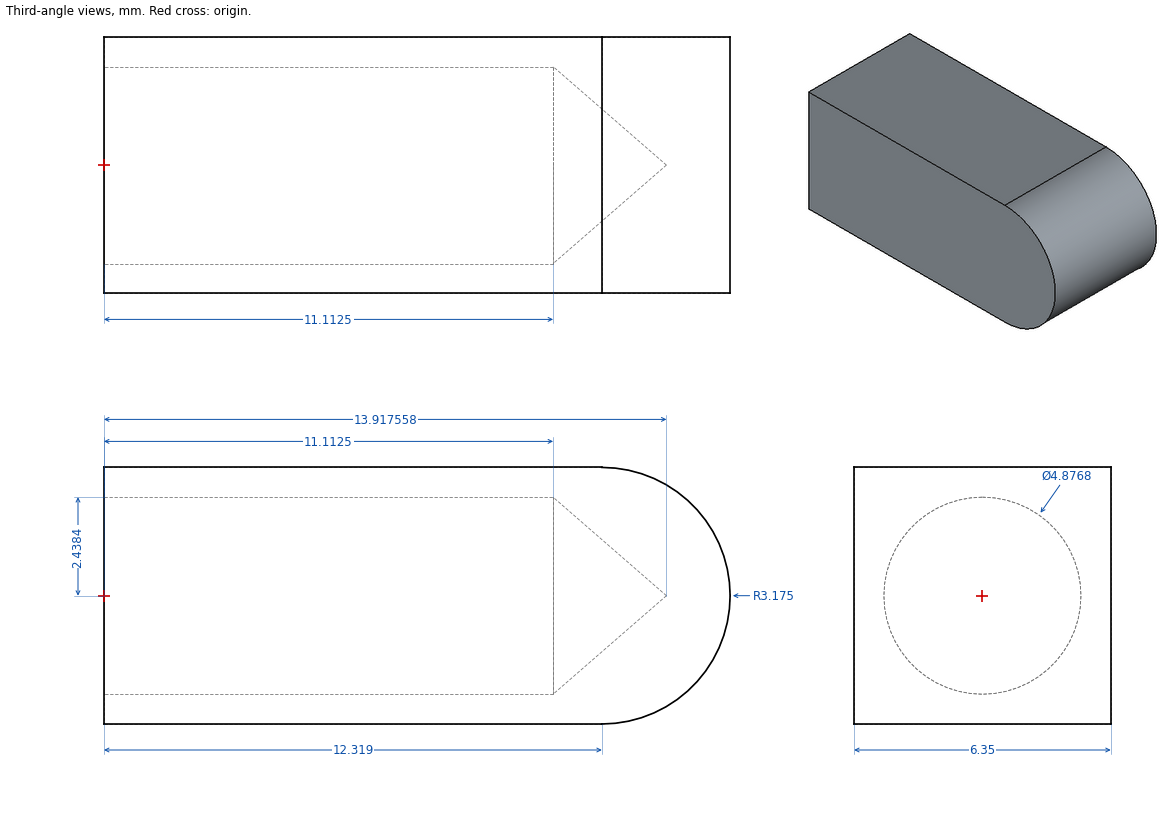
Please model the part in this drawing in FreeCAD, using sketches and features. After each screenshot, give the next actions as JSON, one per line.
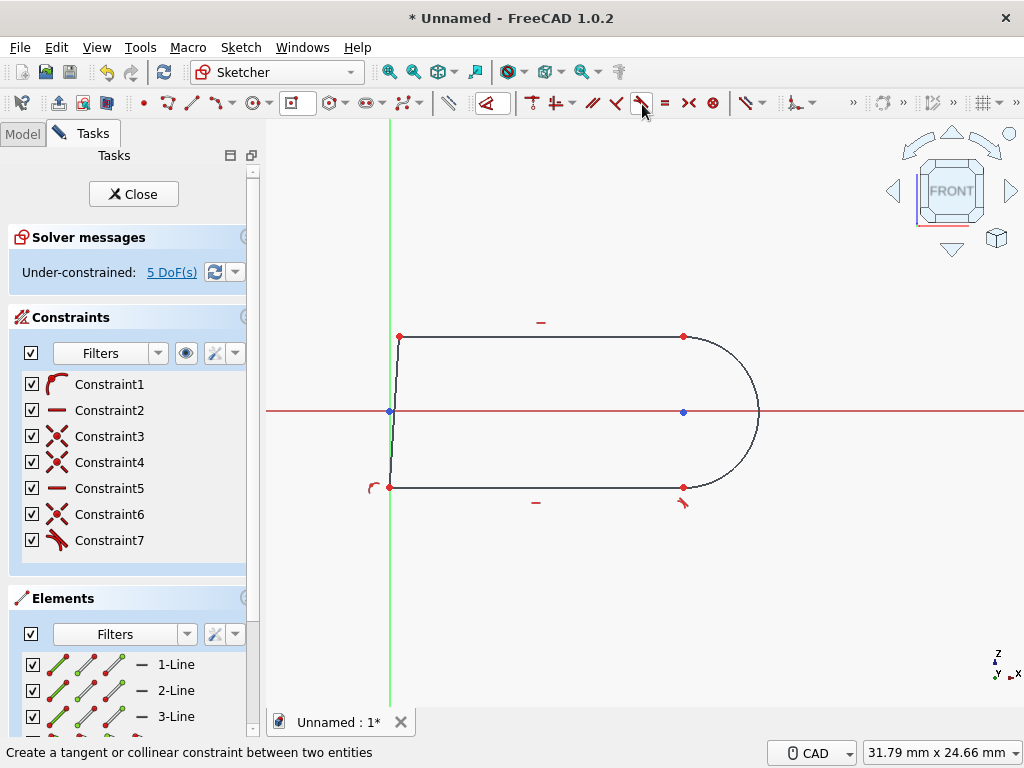
{"action": "left_click", "coordinate": [484, 337]}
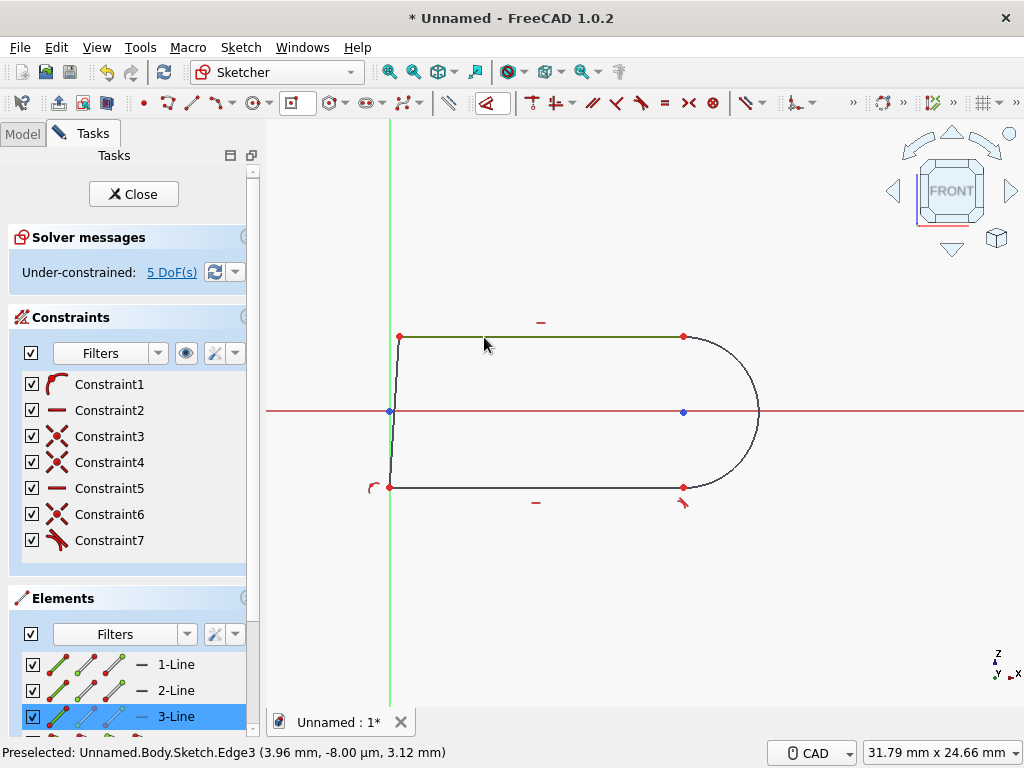
{"action": "left_click", "coordinate": [744, 457]}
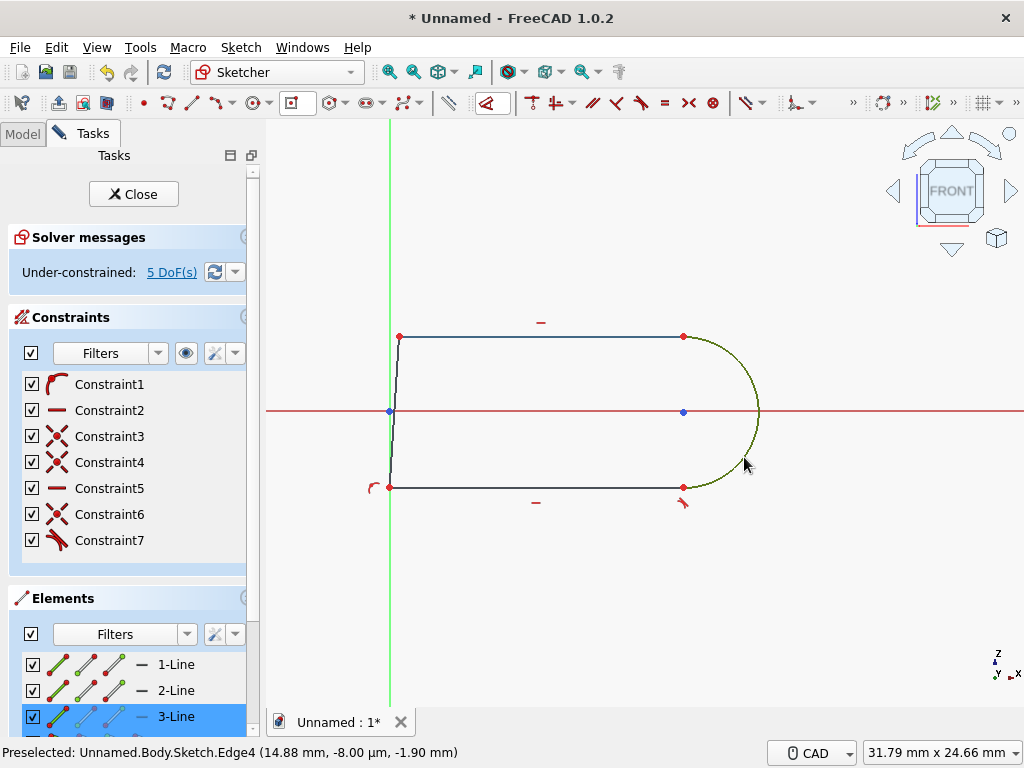
{"action": "key", "text": "t"}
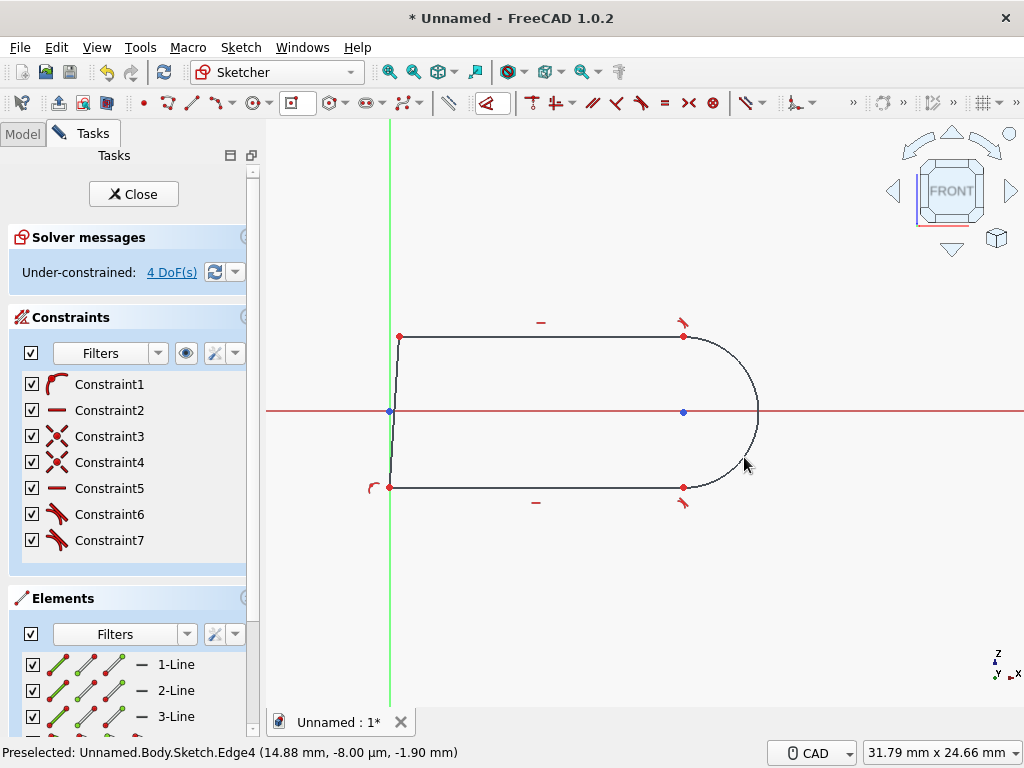
{"action": "left_click", "coordinate": [392, 443]}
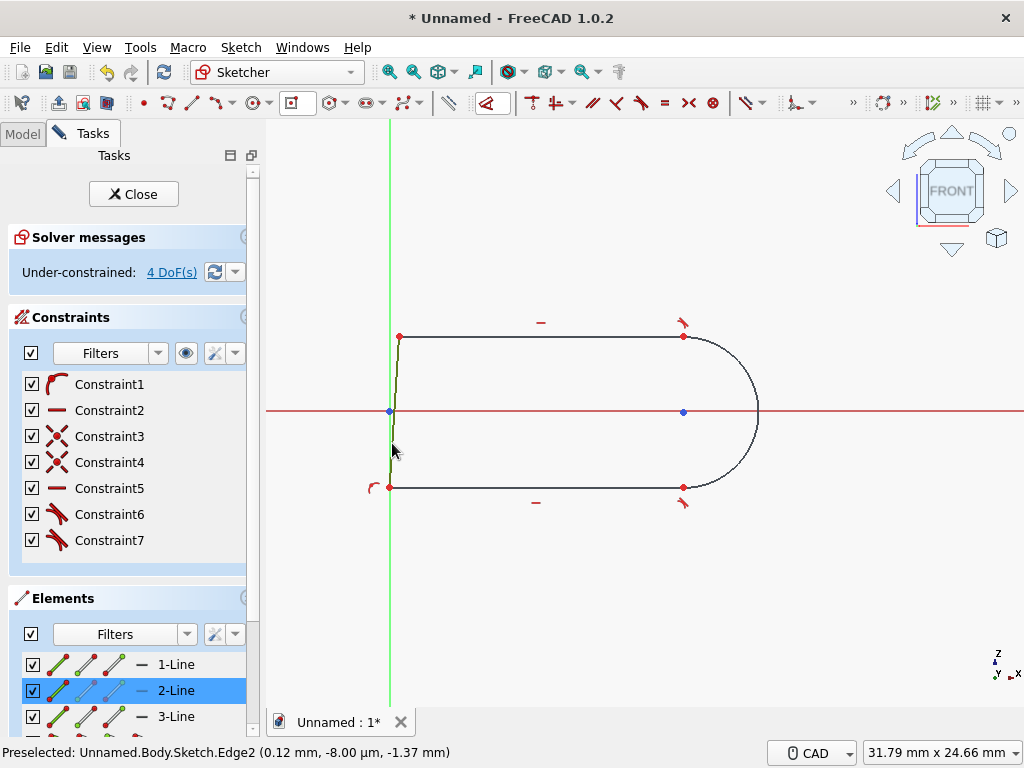
{"action": "key", "text": "v"}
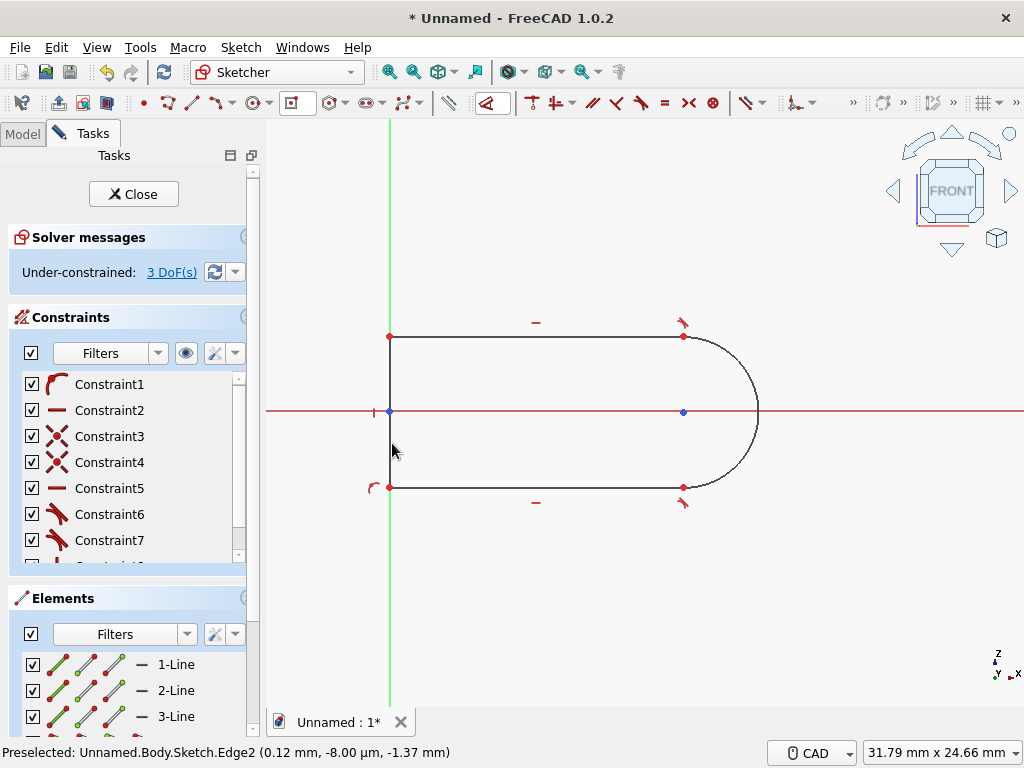
{"action": "left_click", "coordinate": [683, 412]}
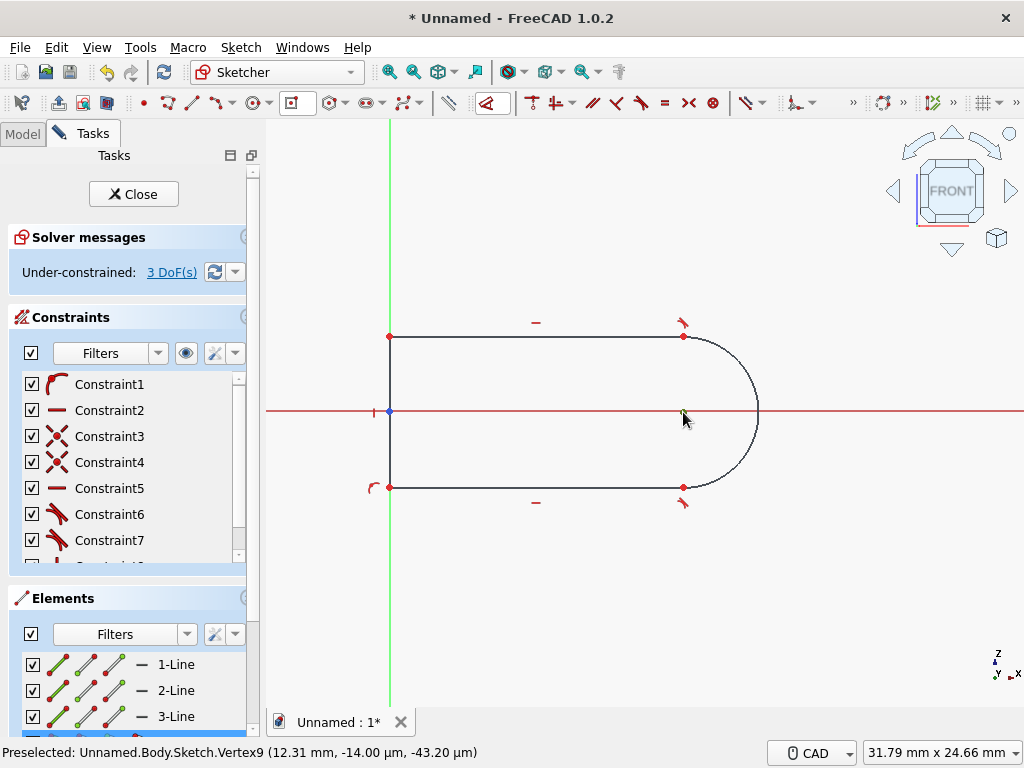
{"action": "left_click", "coordinate": [334, 411]}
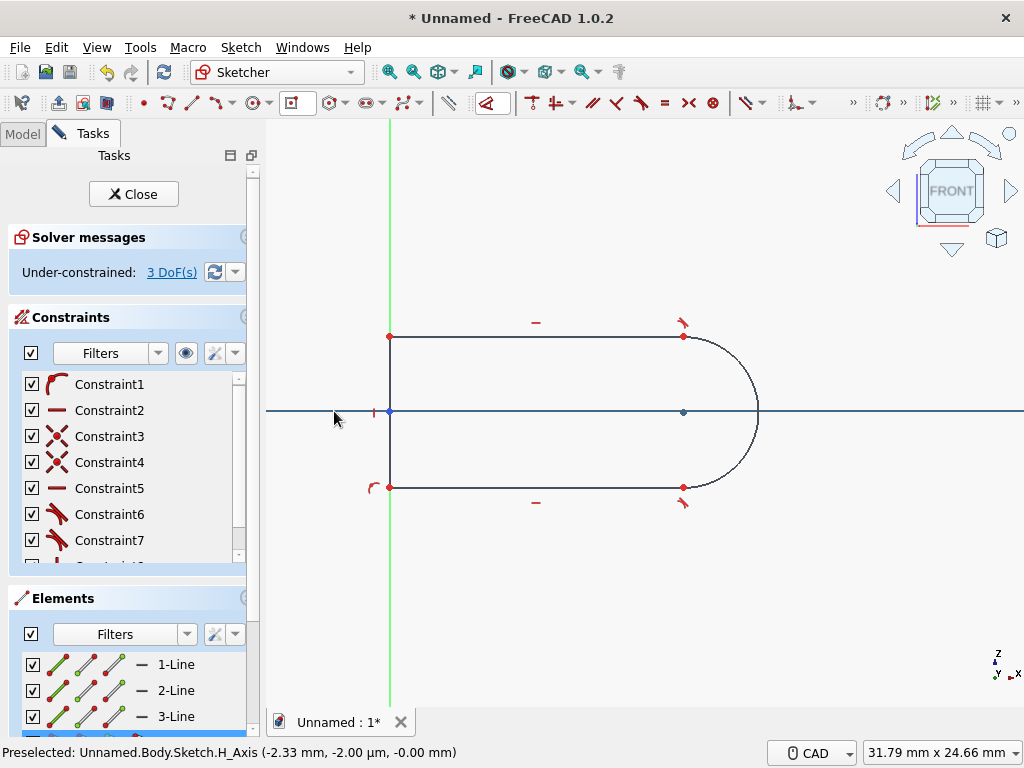
{"action": "key", "text": "c"}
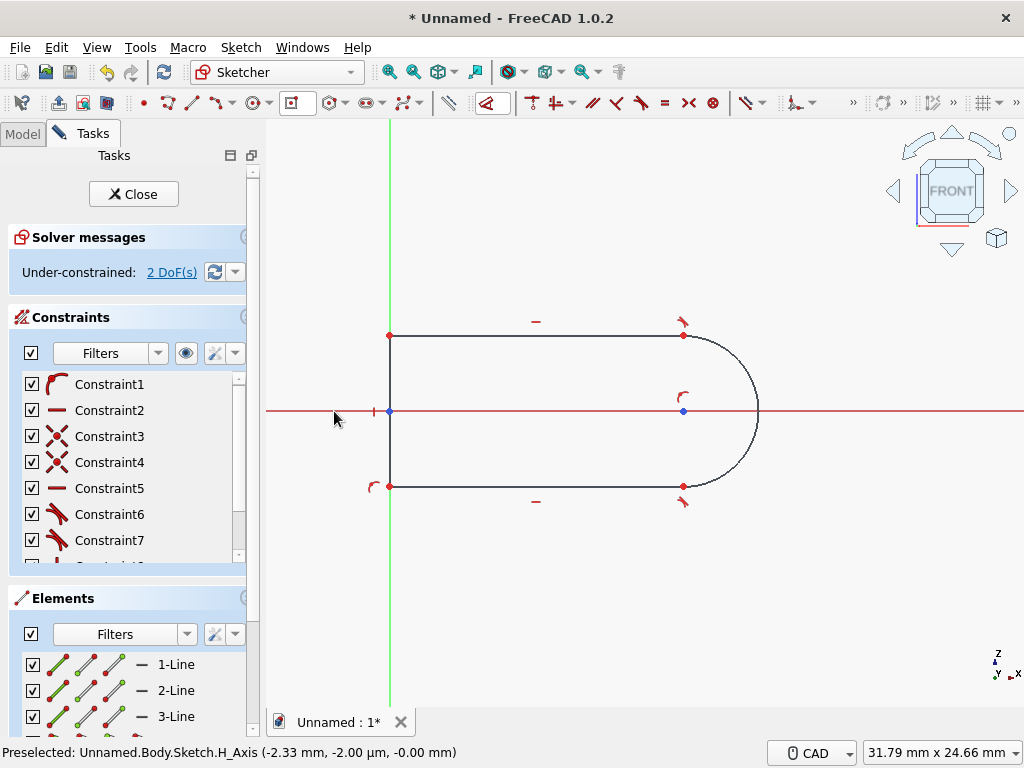
{"action": "key", "text": "d"}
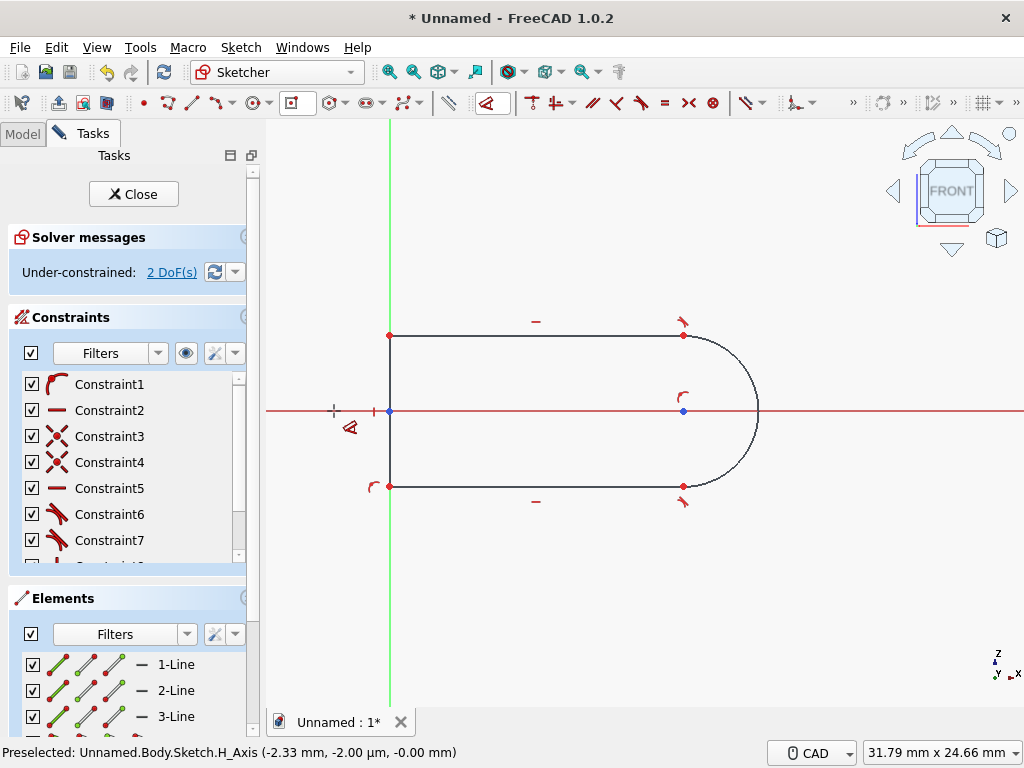
{"action": "left_click", "coordinate": [744, 456]}
{"action": "left_click", "coordinate": [770, 475]}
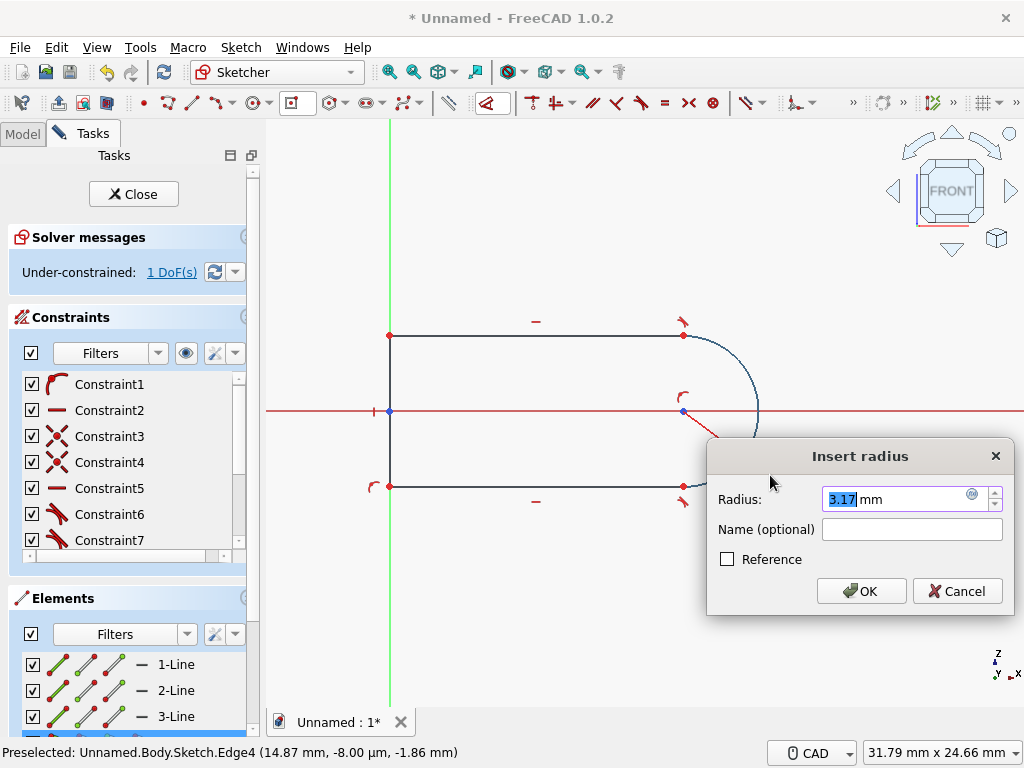
{"action": "type", "text": "3.175"}
{"action": "key", "text": "Return"}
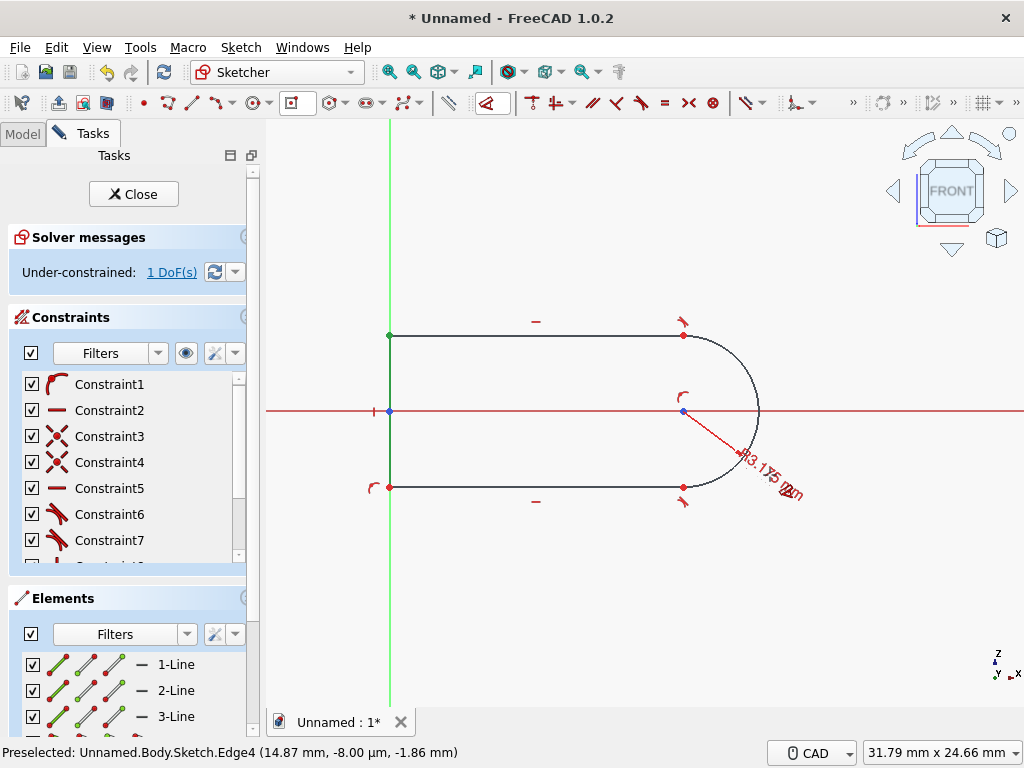
{"action": "left_click", "coordinate": [595, 487]}
{"action": "left_click", "coordinate": [536, 521]}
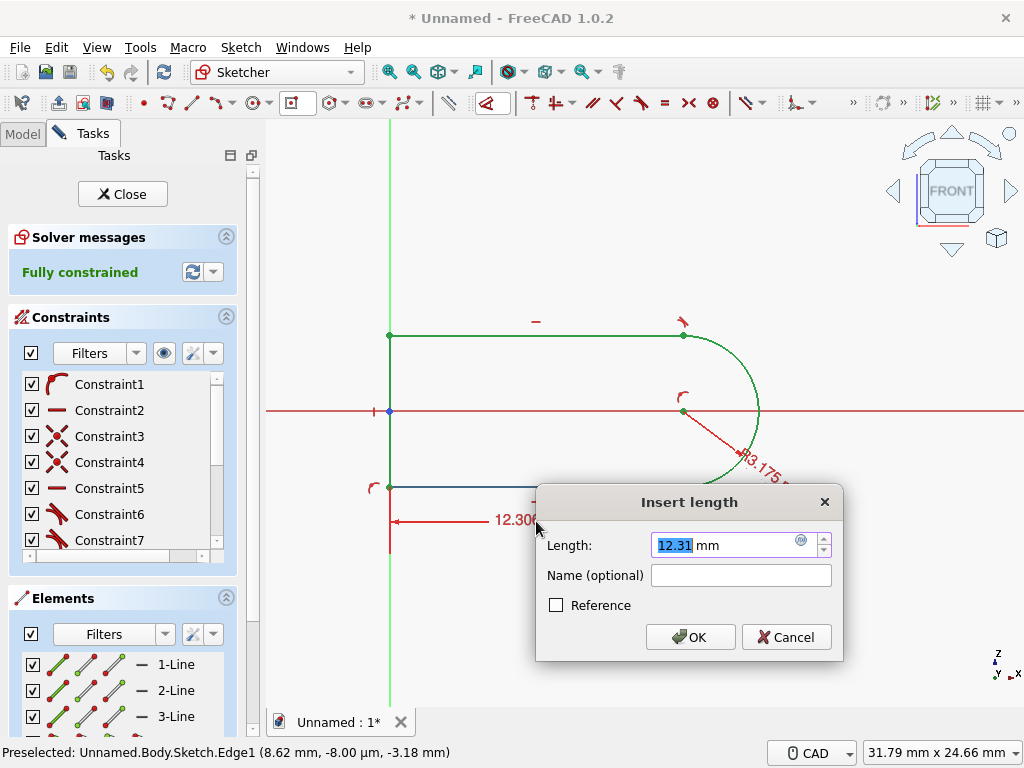
{"action": "type", "text": "12.319"}
{"action": "key", "text": "Return"}
{"action": "key", "text": "Escape"}